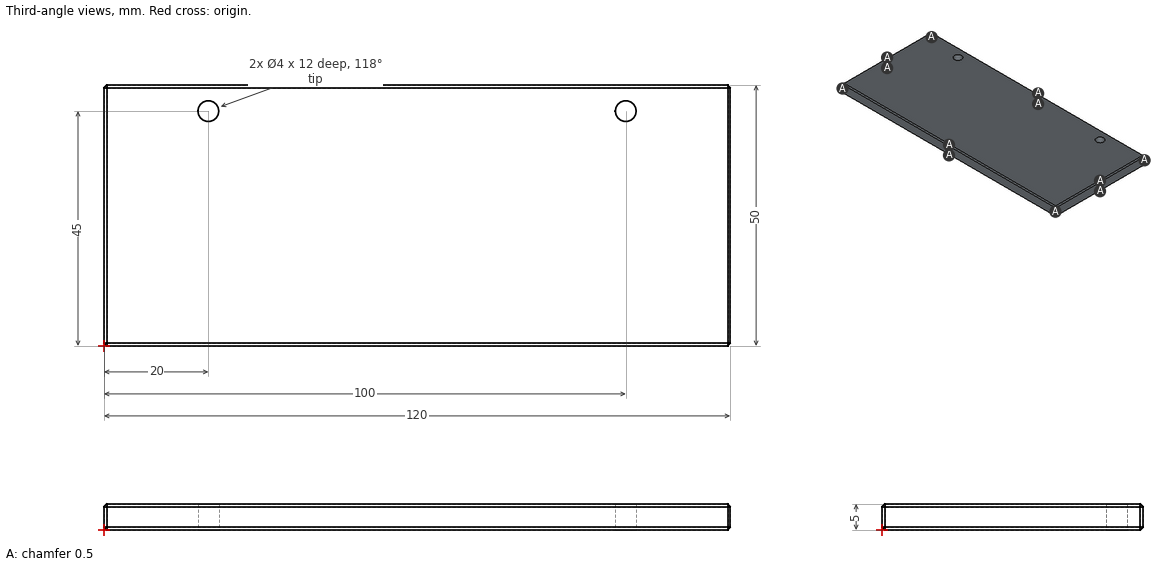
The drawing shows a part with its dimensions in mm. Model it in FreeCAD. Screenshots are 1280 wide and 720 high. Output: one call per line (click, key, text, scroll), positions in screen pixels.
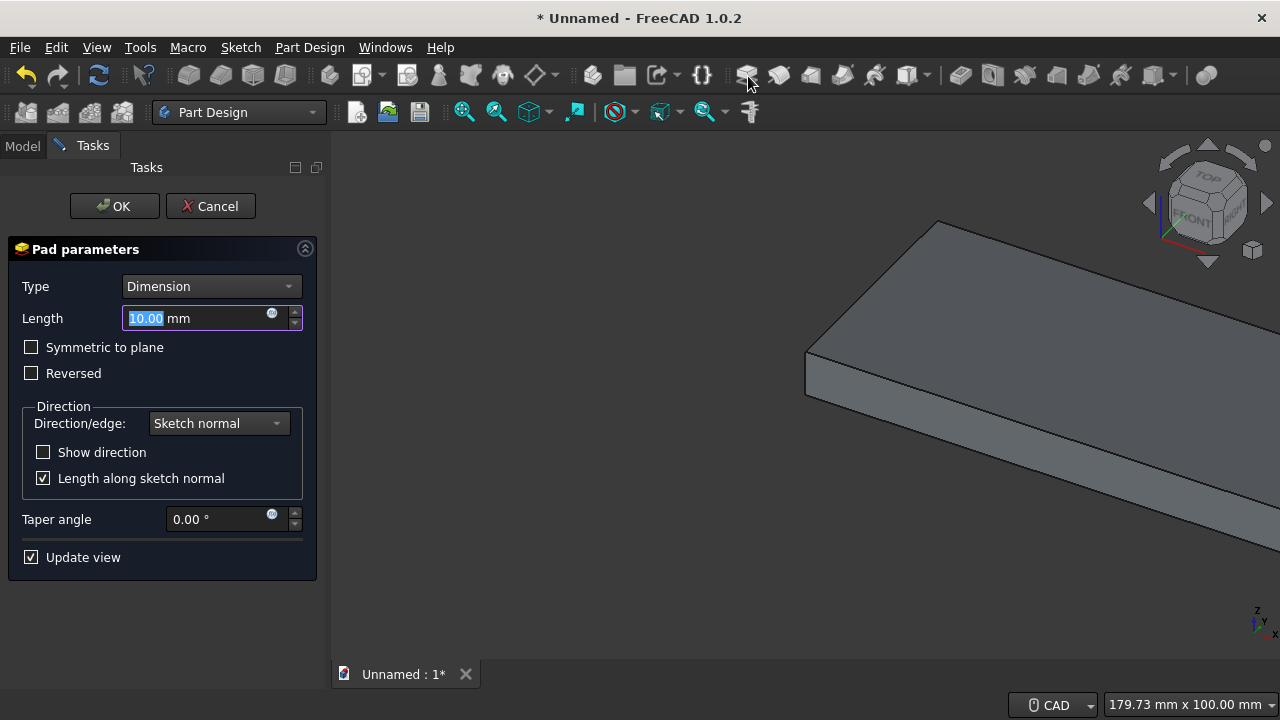
text(5)
key(Tab)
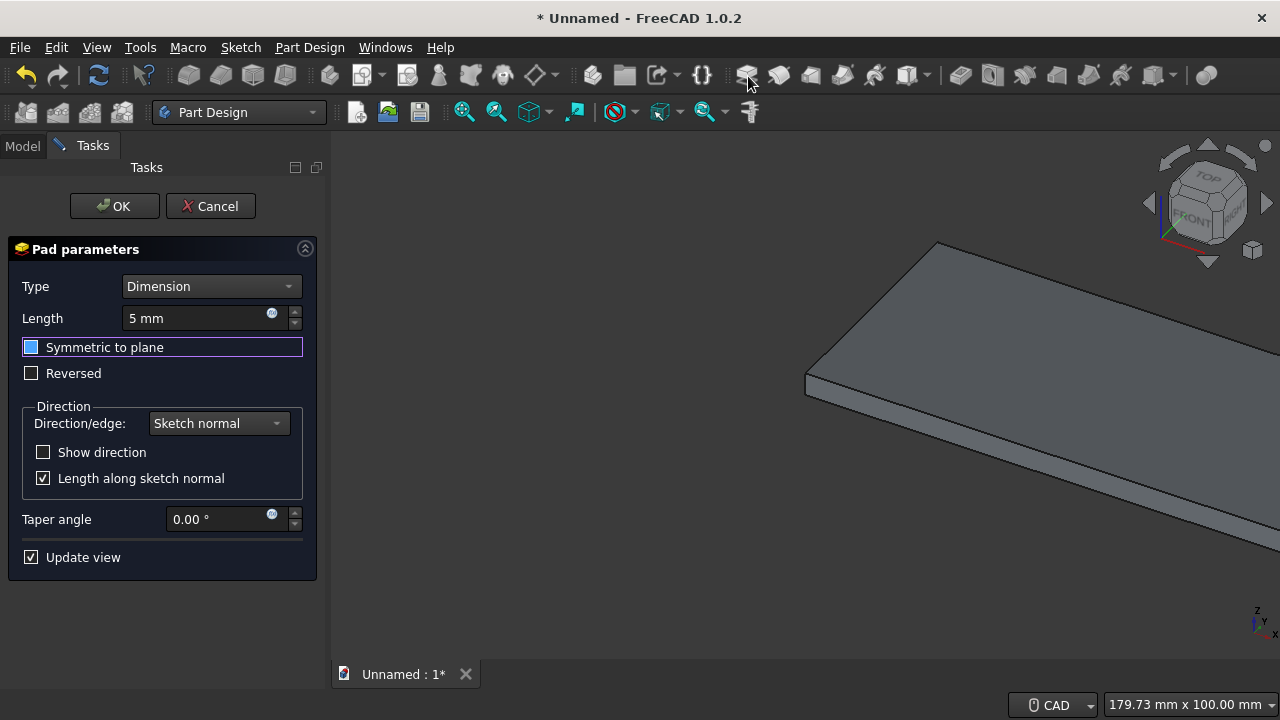
click(115, 206)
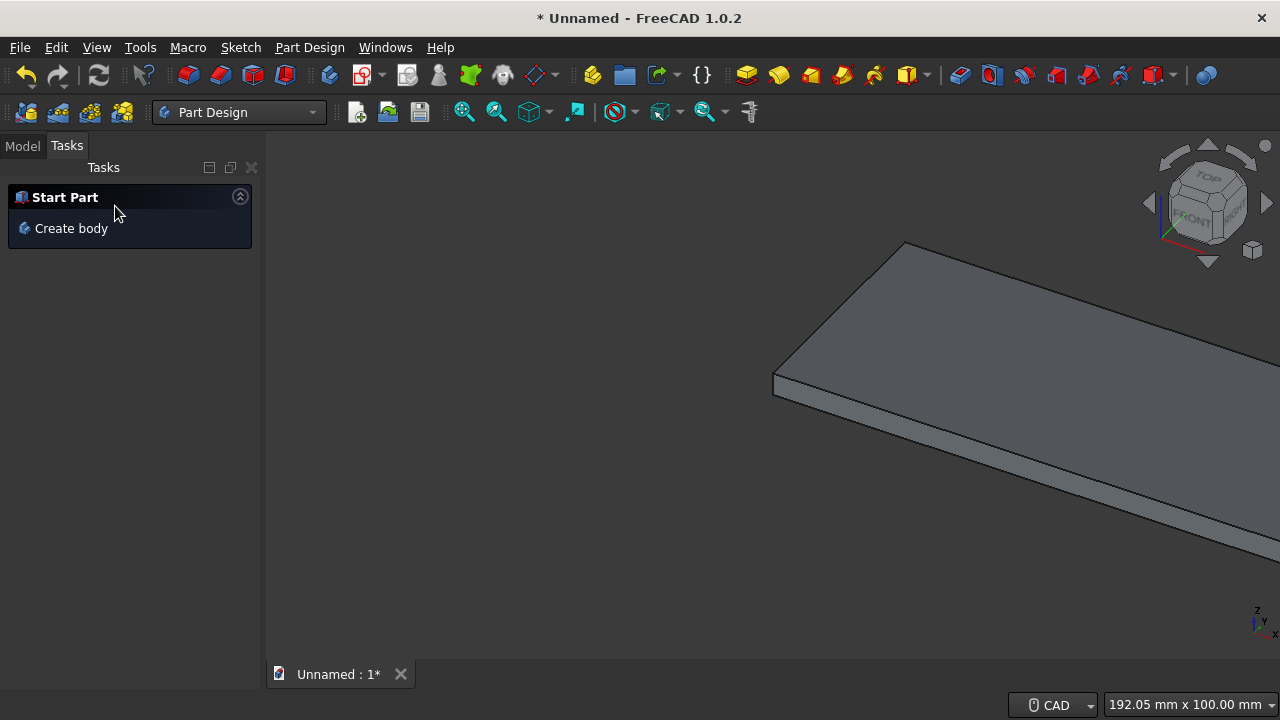
click(466, 112)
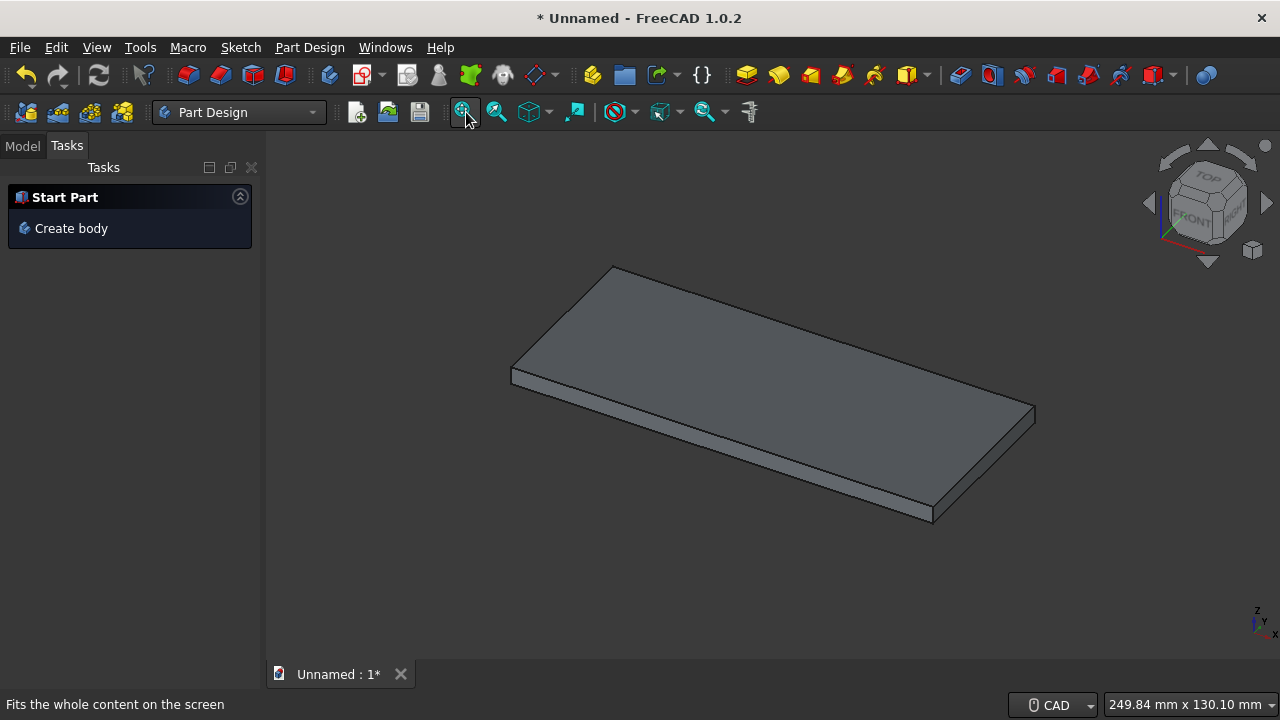
click(894, 426)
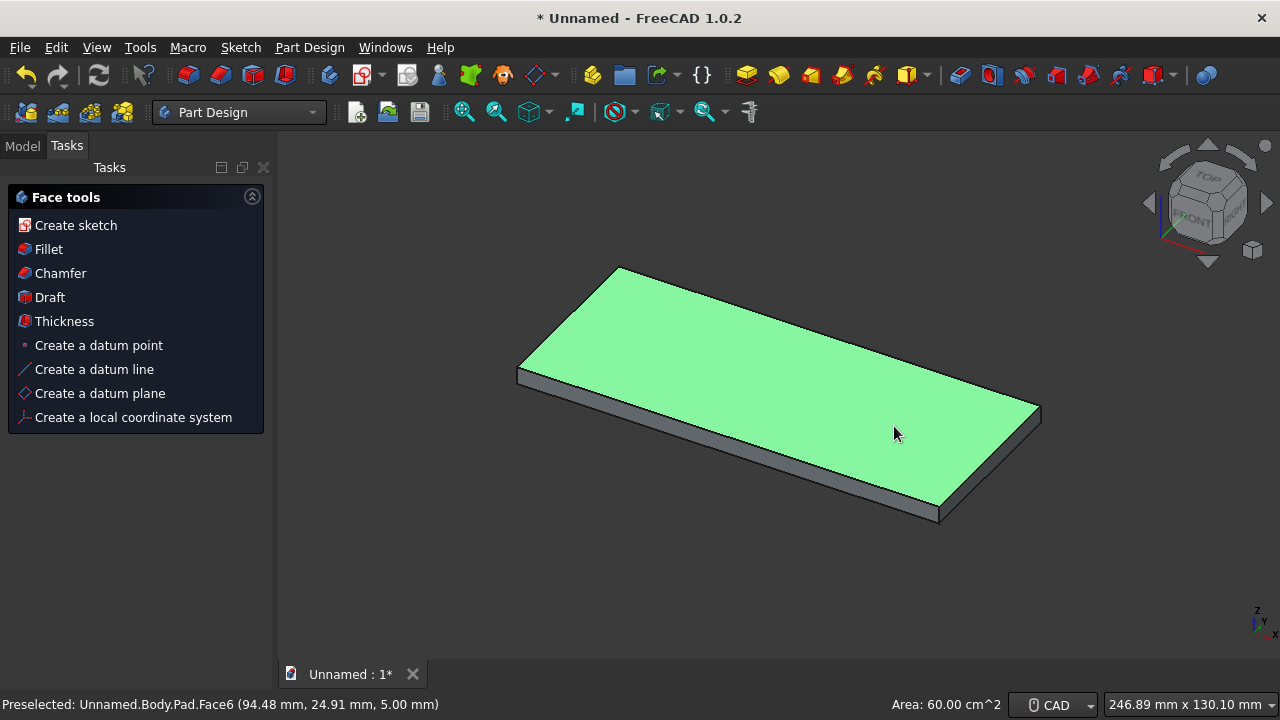
click(362, 76)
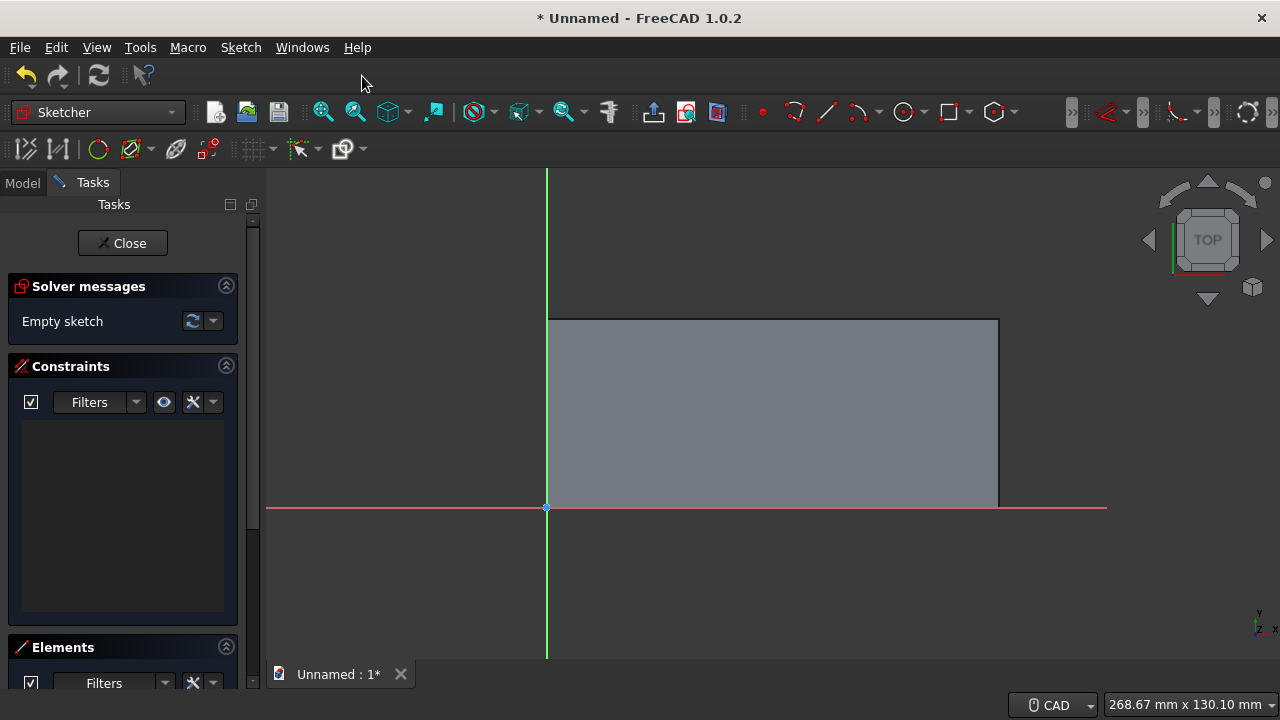
scroll(809, 431, up, 2)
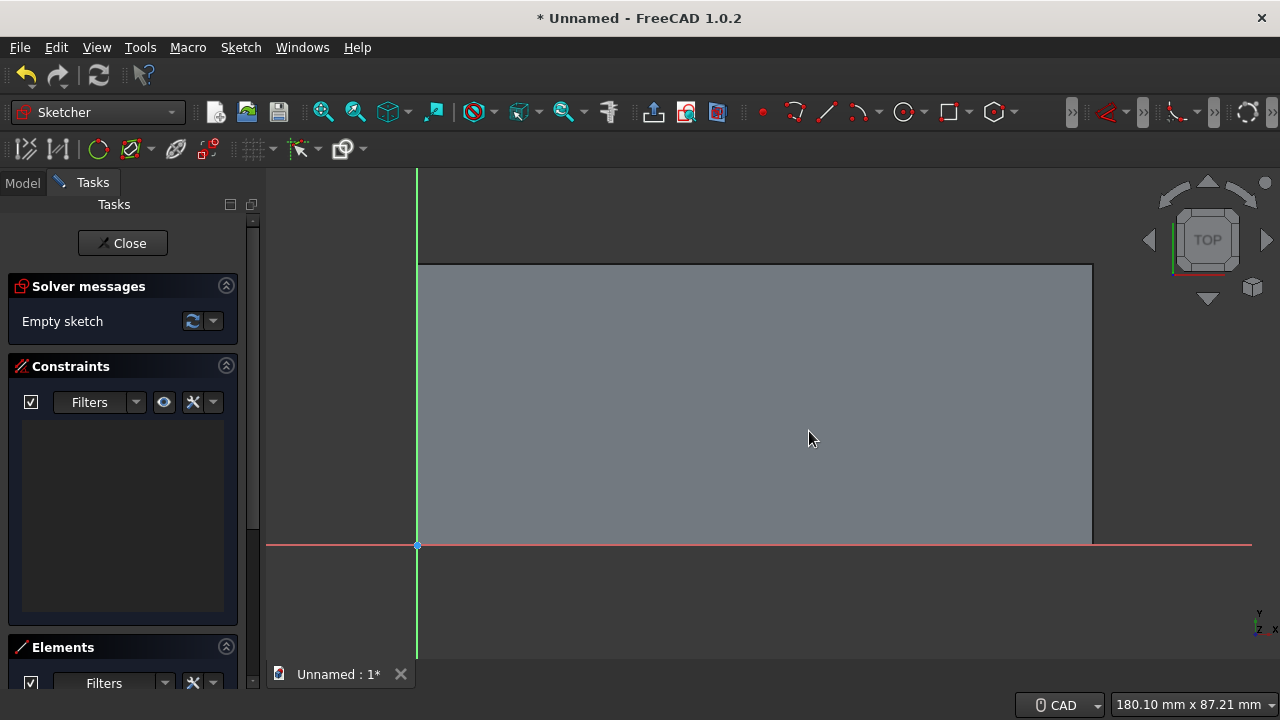
click(904, 112)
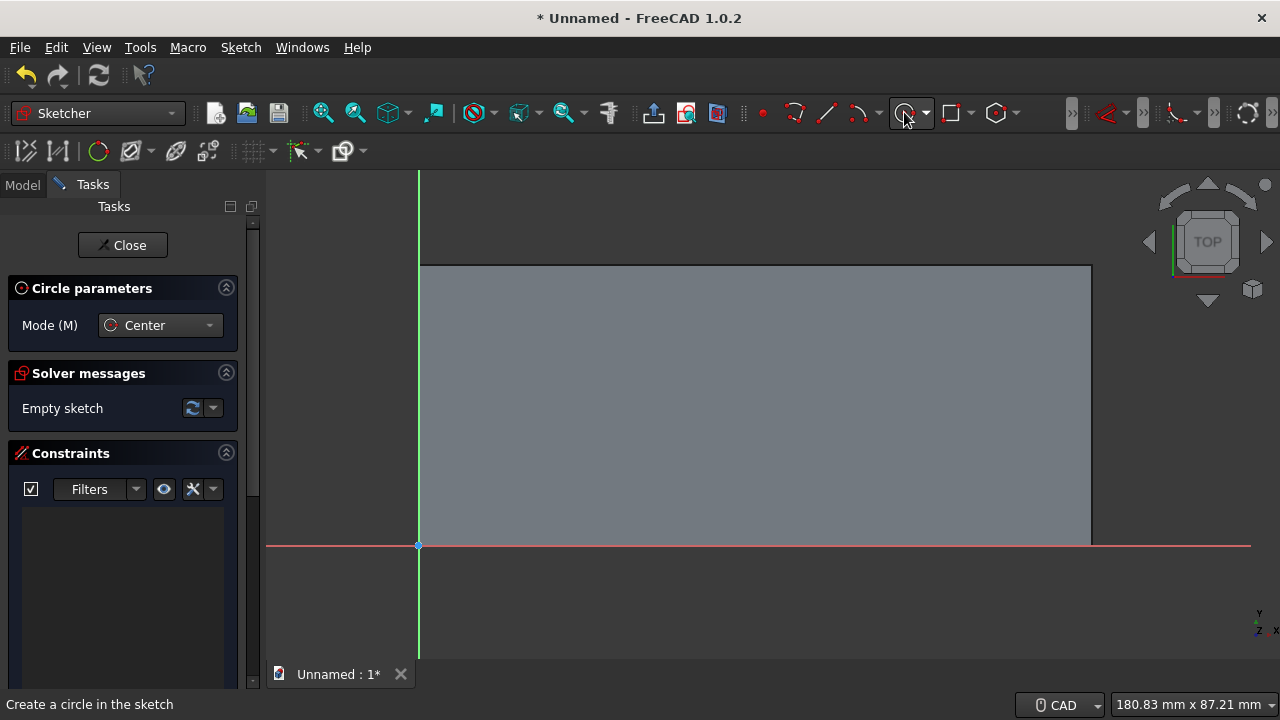
scroll(531, 294, up, 4)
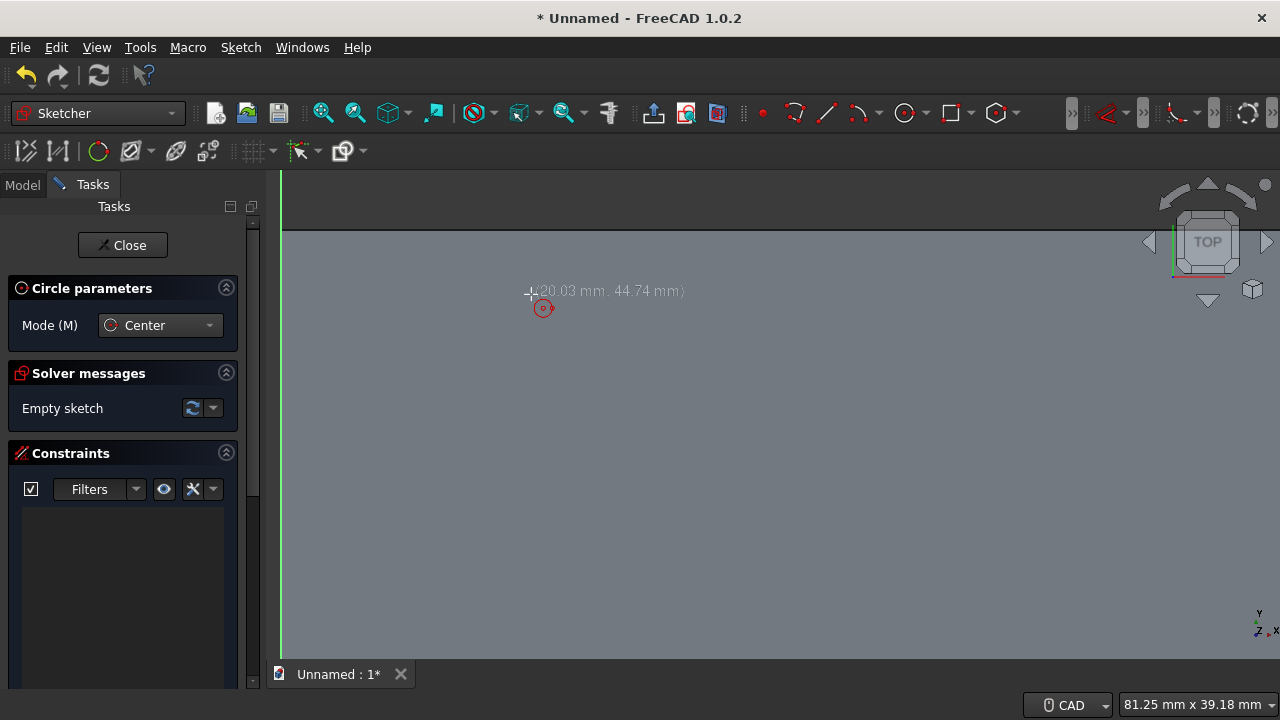
click(530, 293)
move(548, 275)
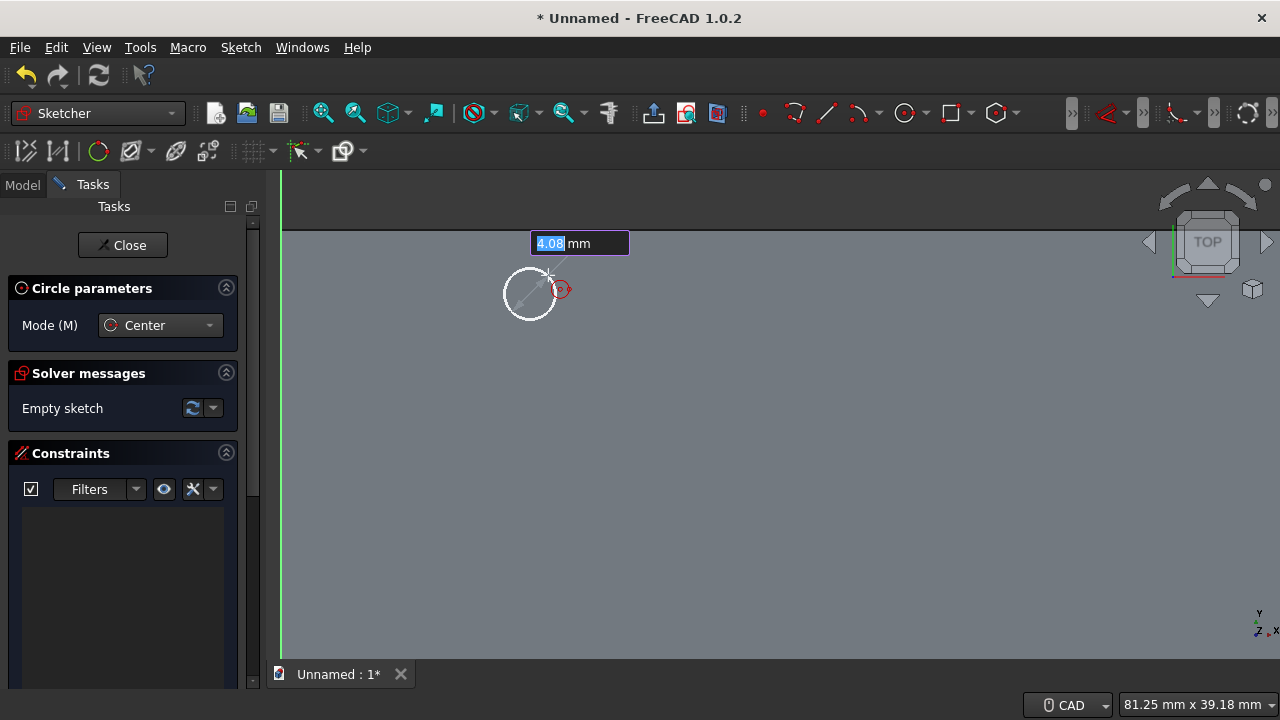
text(4)
key(Return)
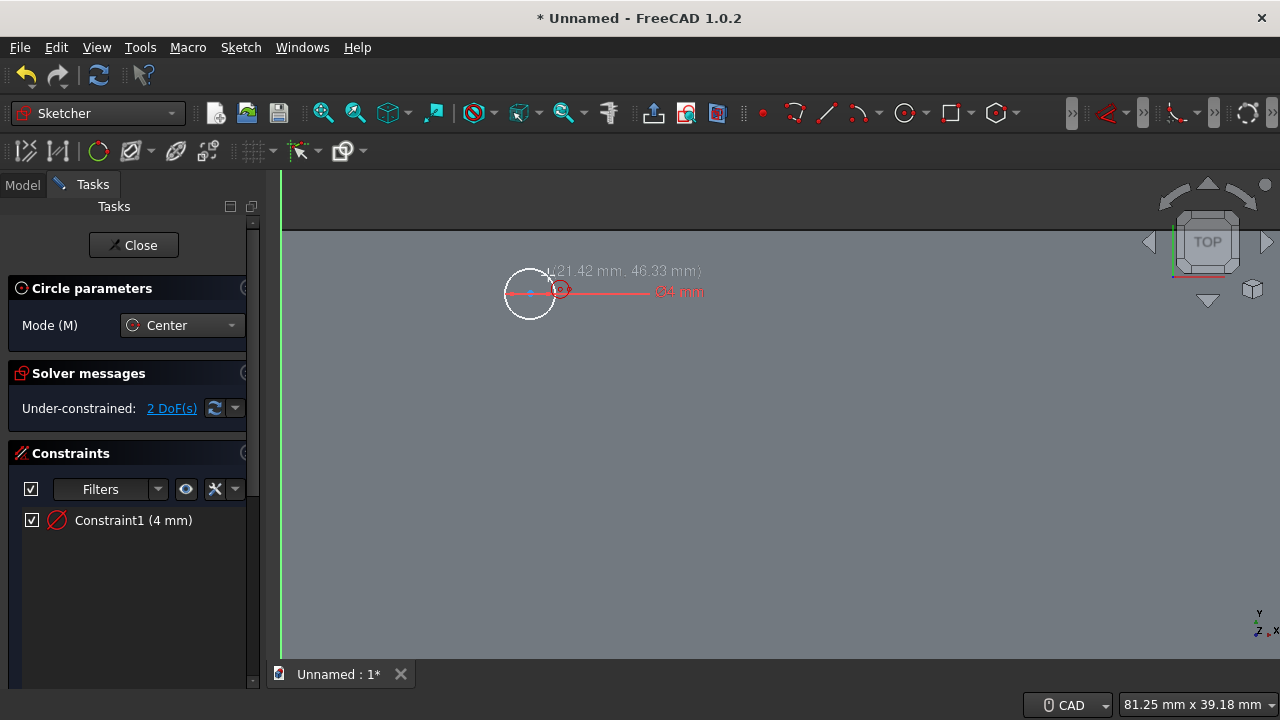
scroll(531, 295, down, 4)